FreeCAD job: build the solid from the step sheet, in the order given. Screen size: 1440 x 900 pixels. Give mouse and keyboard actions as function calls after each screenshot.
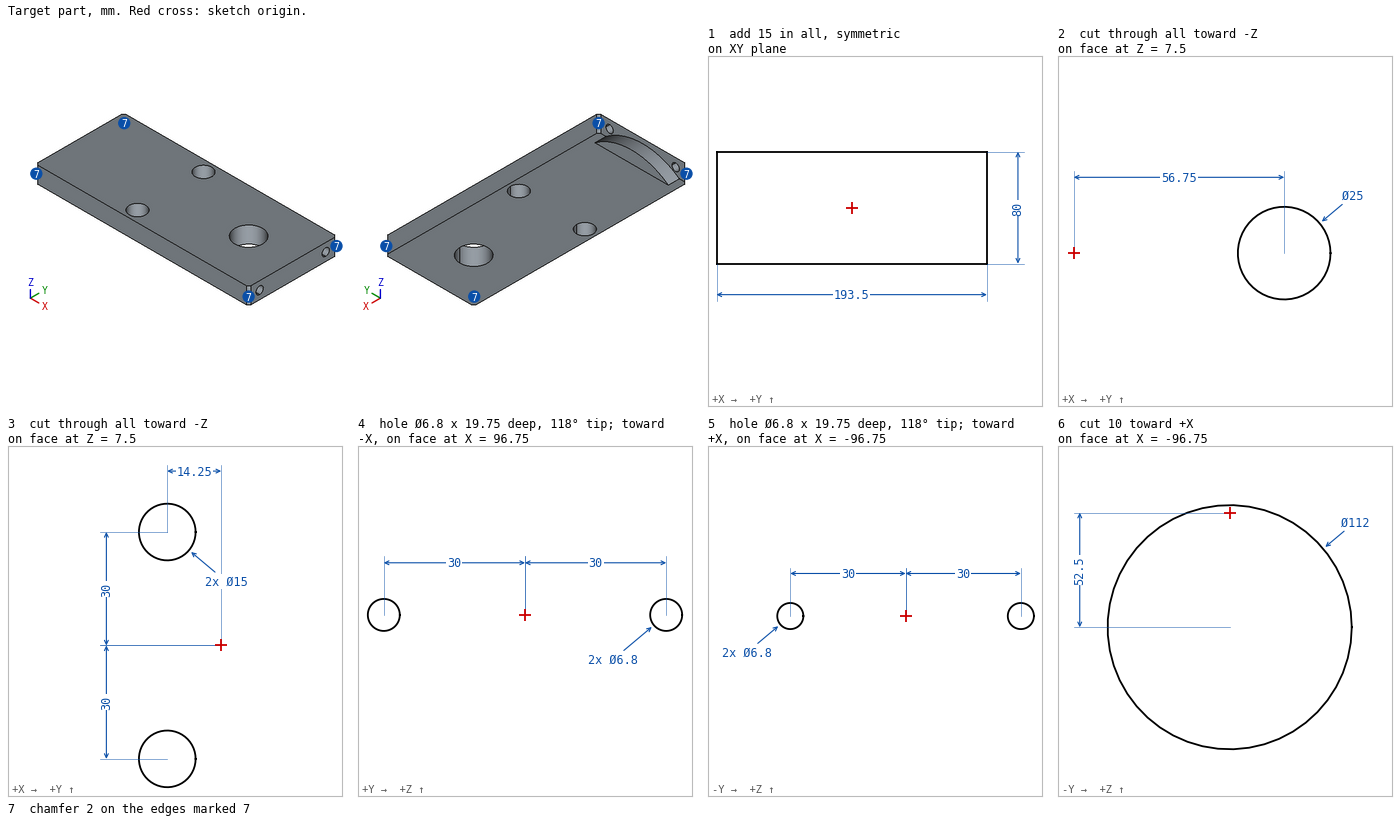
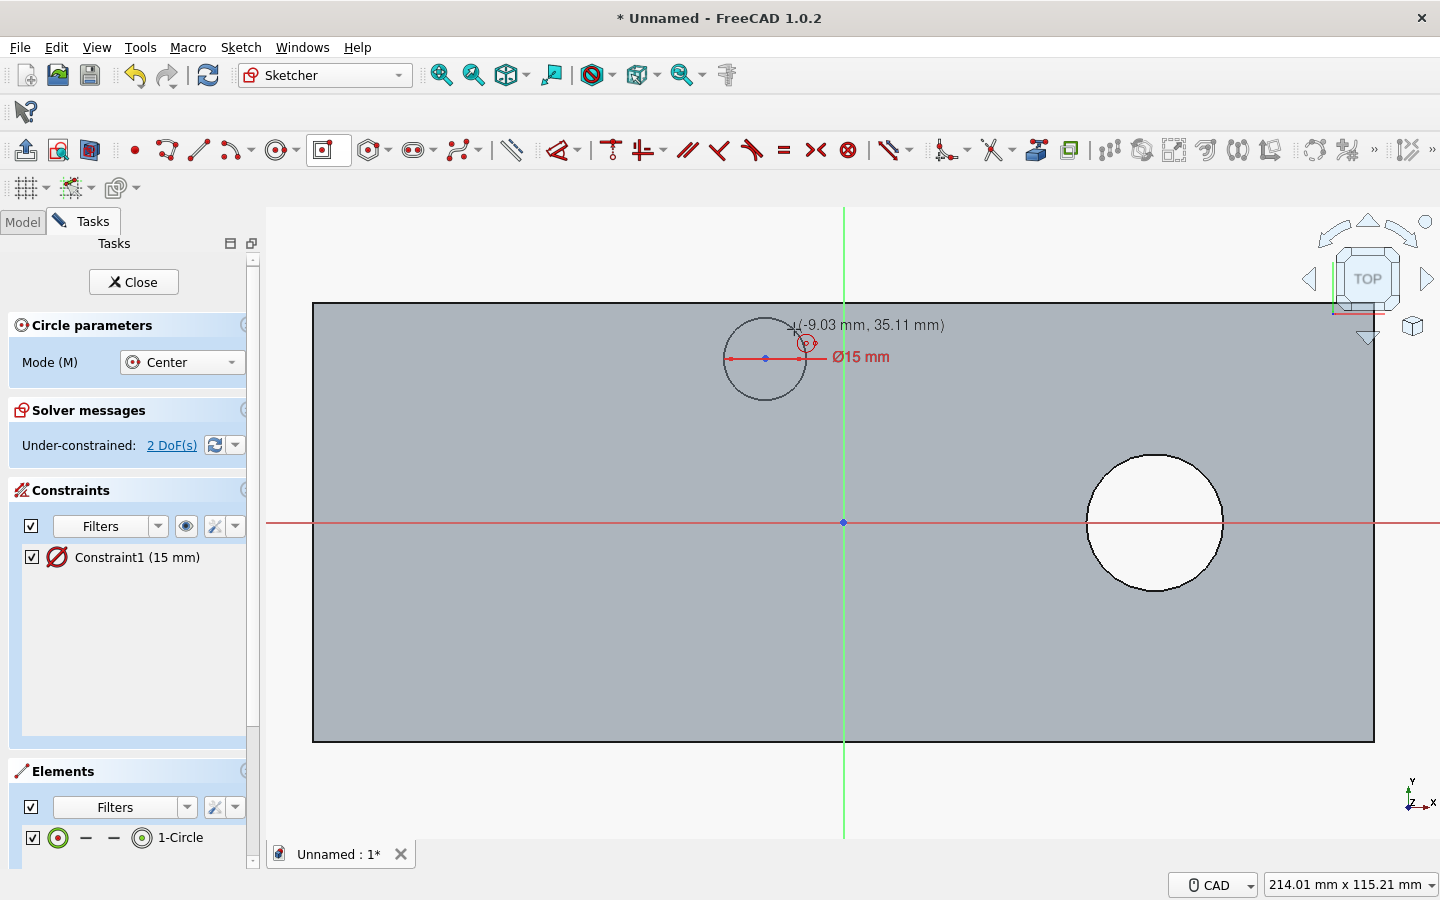
click(765, 687)
move(794, 658)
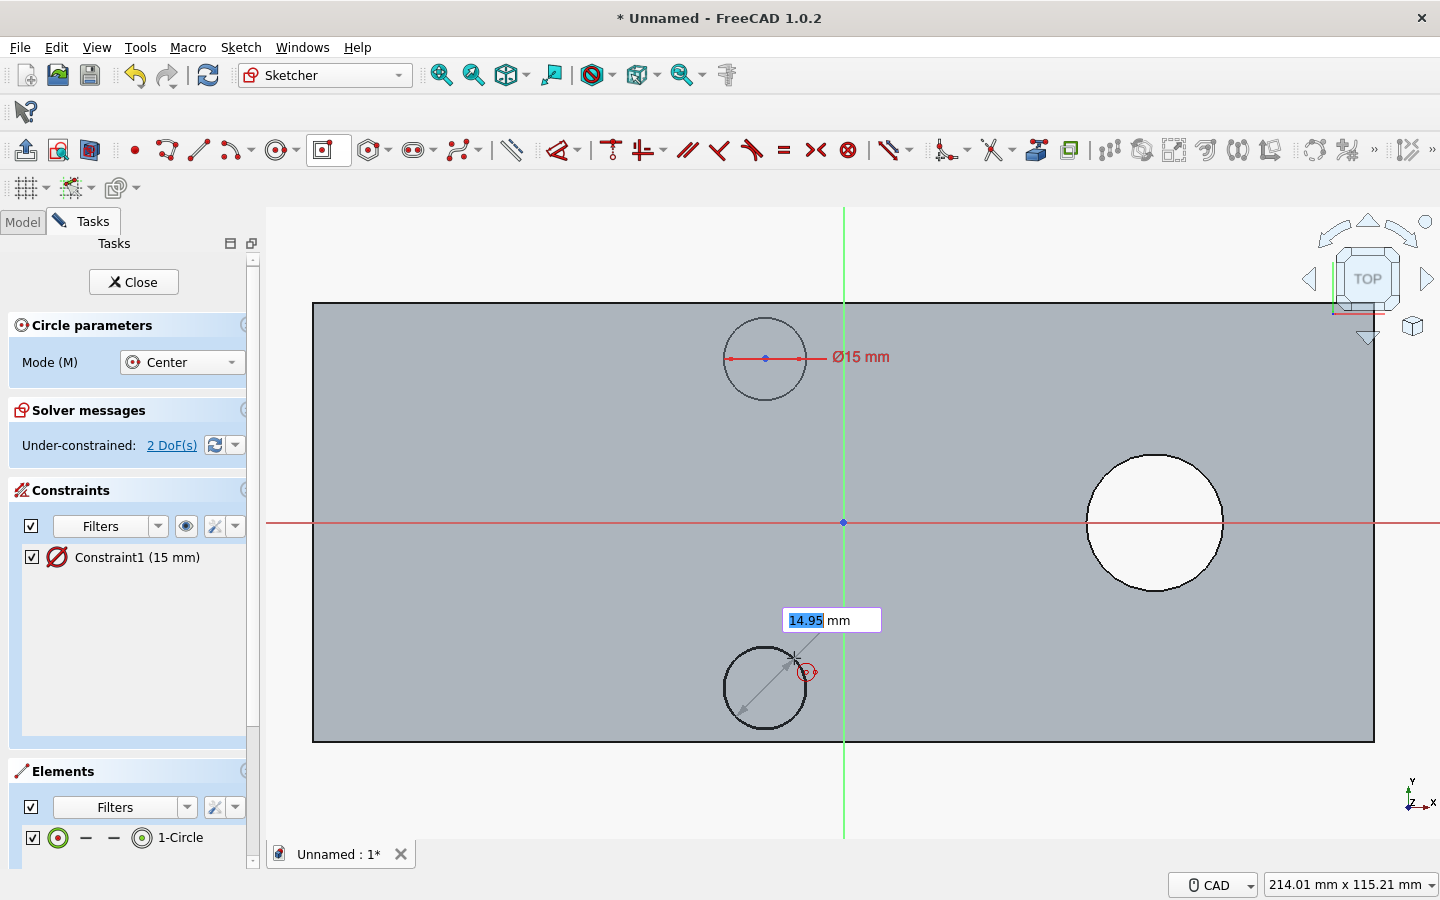
text(15)
key(Return)
key(Escape)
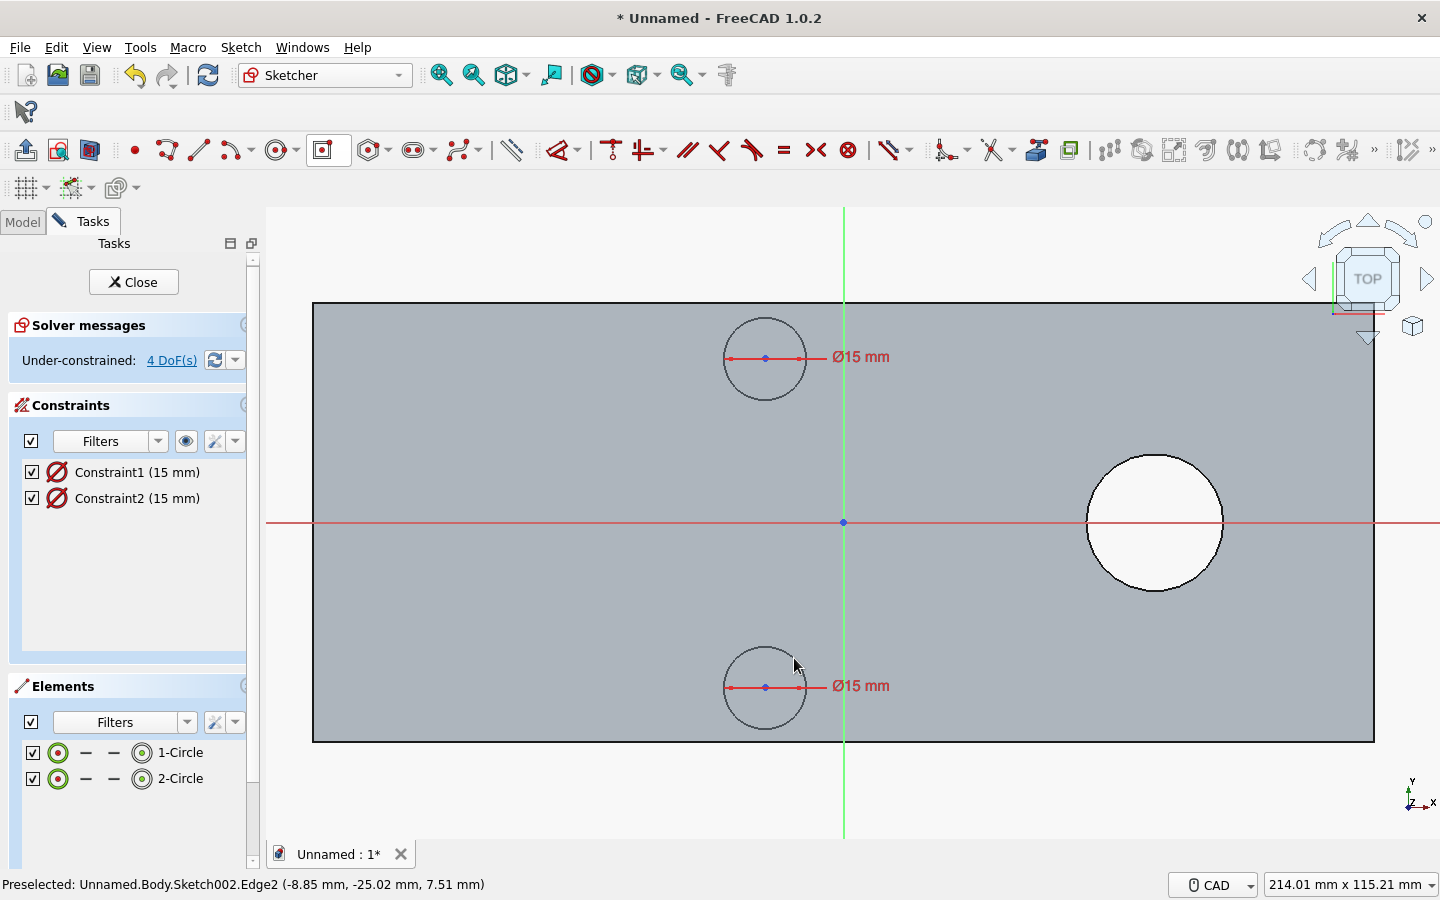
click(765, 359)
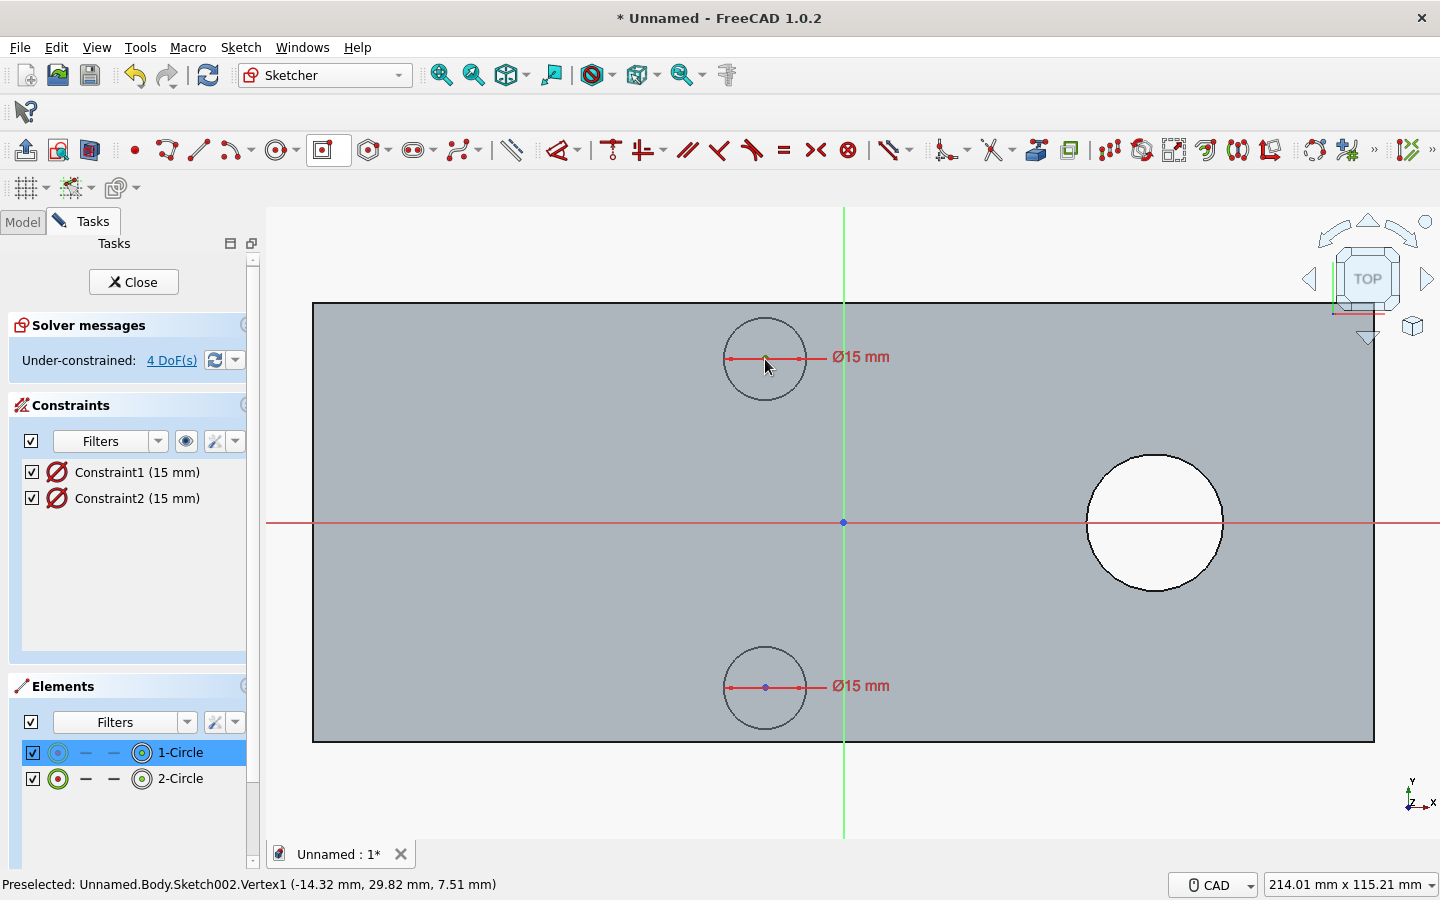
click(765, 688)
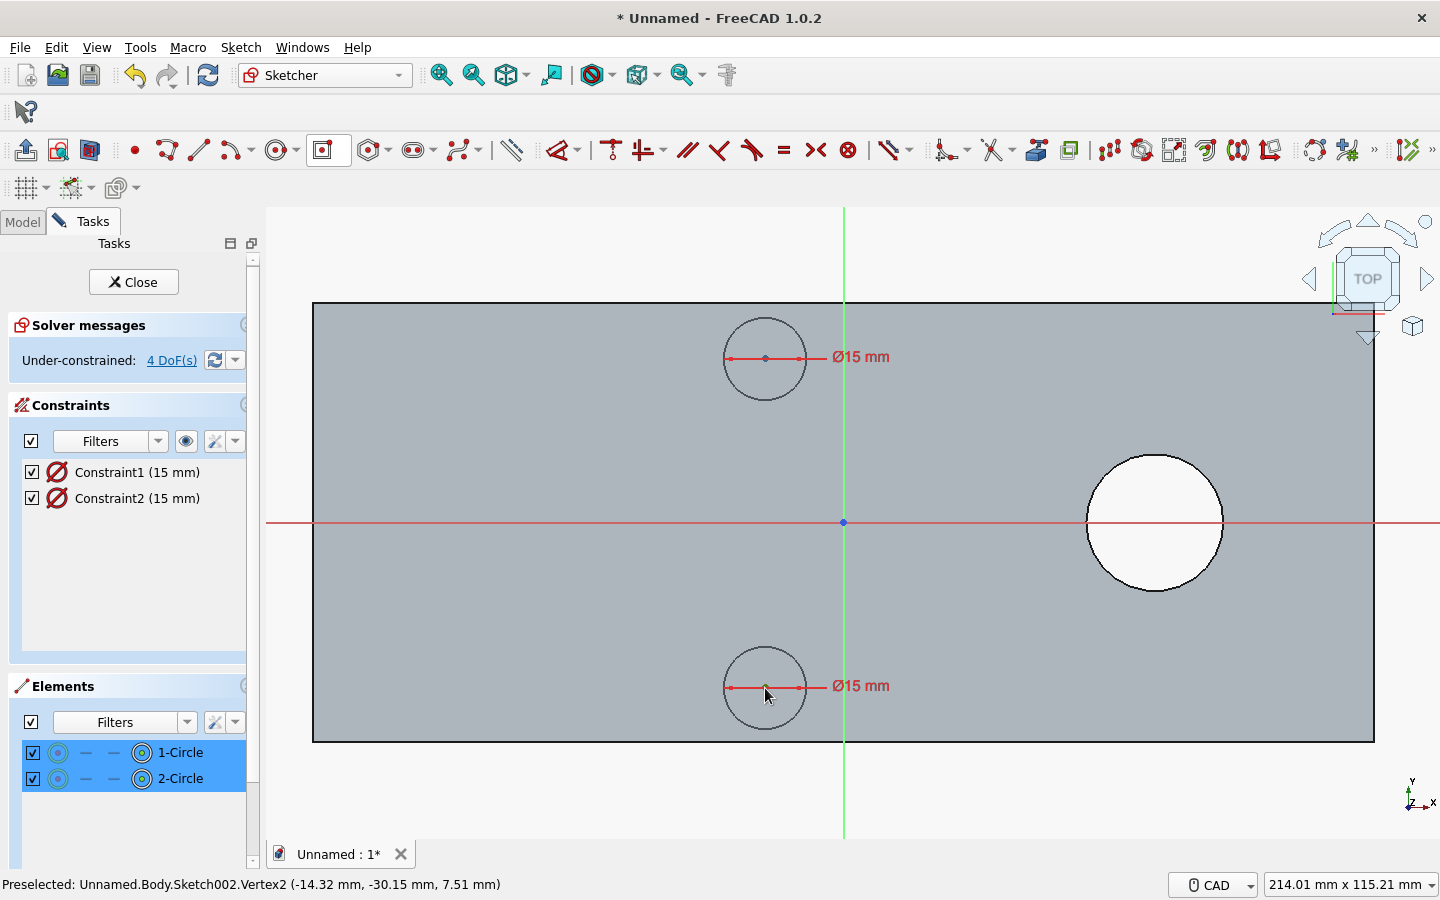
click(666, 150)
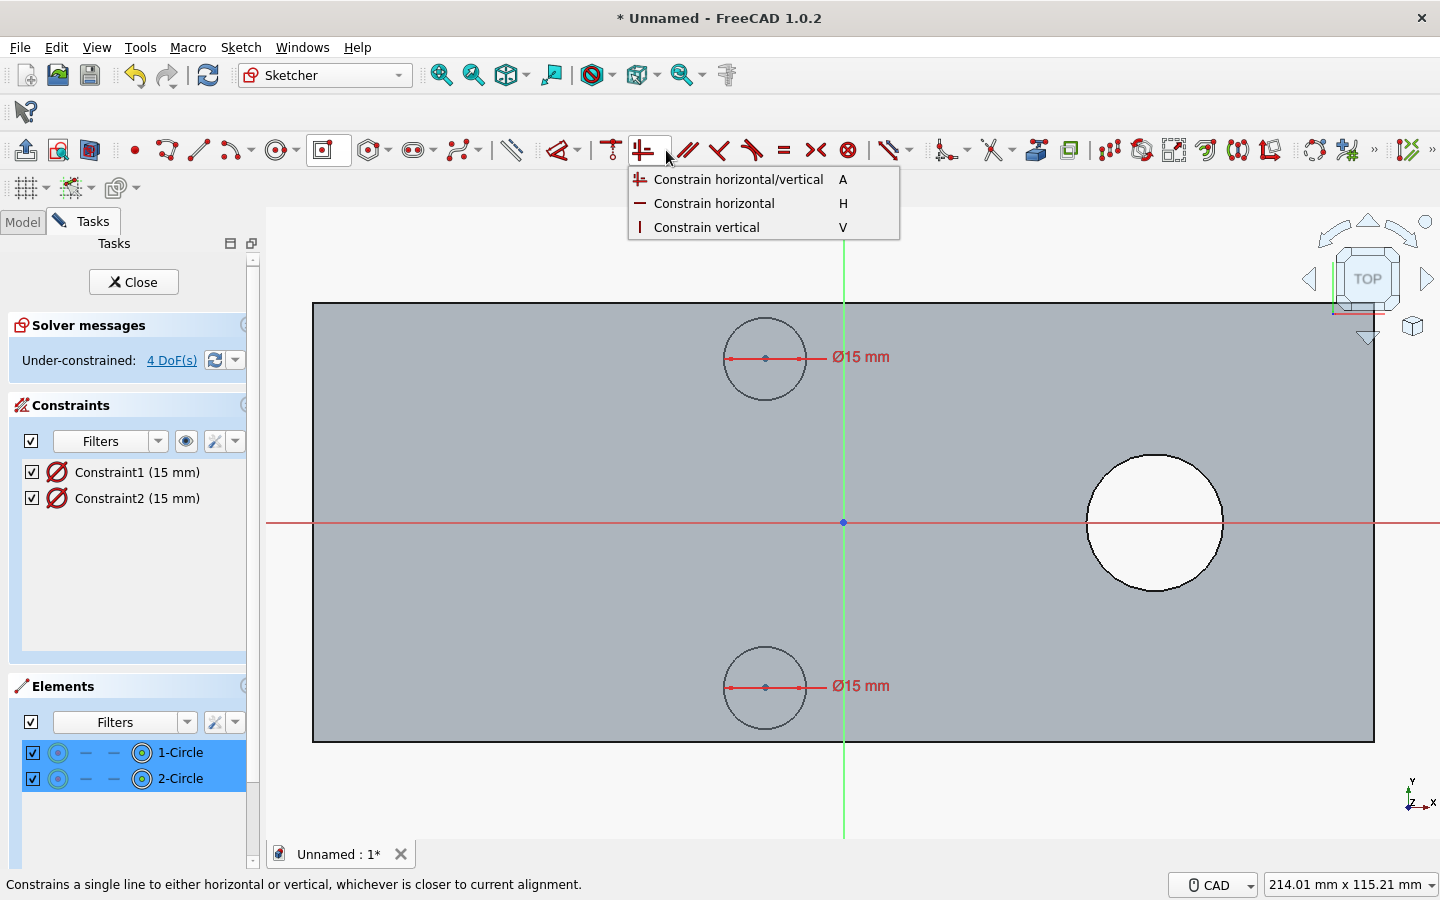
click(764, 227)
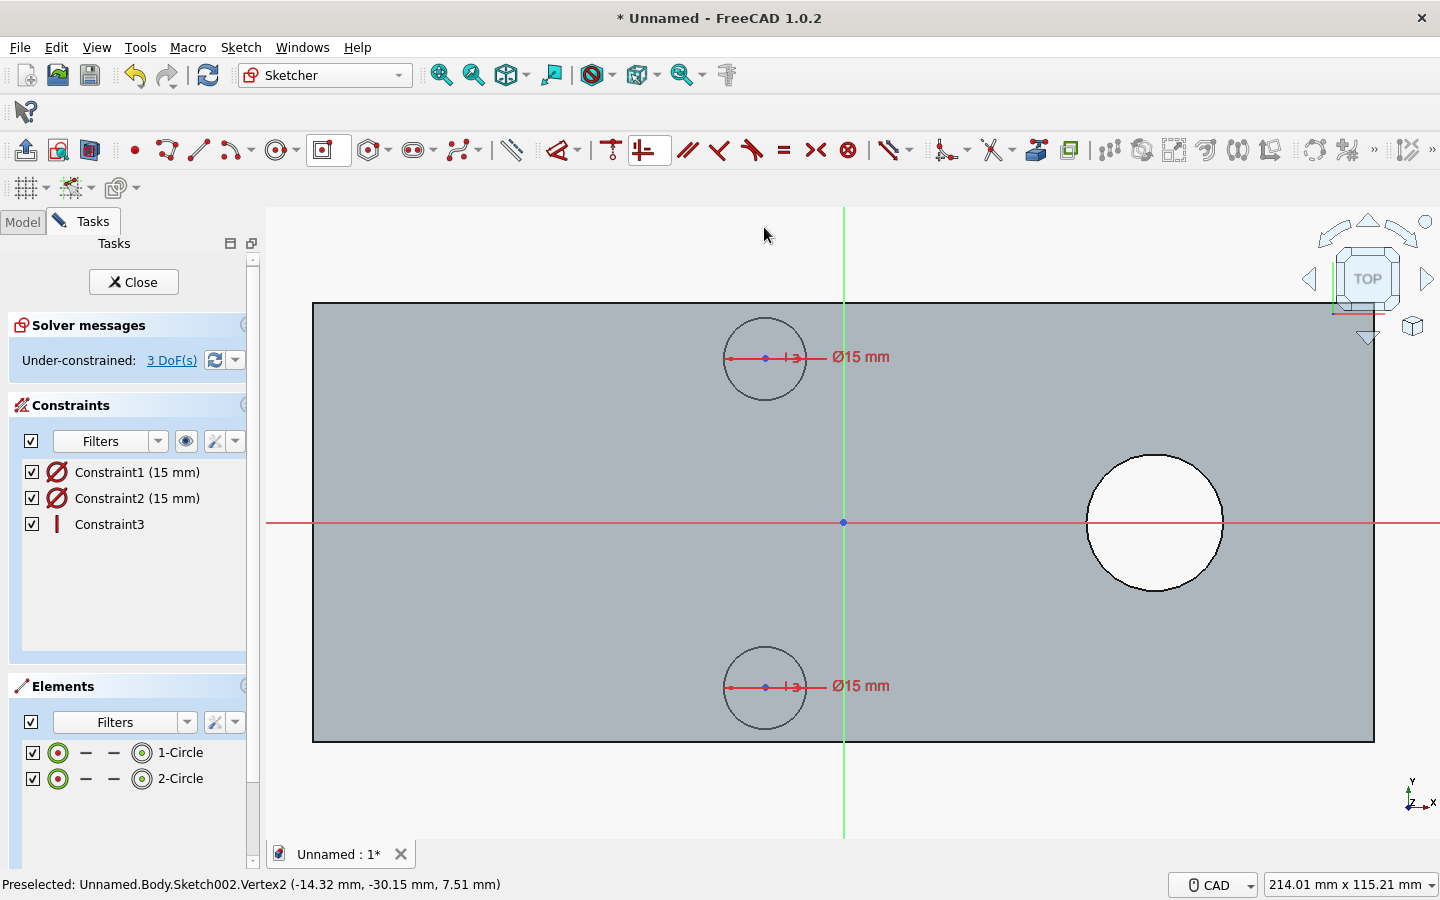
click(765, 359)